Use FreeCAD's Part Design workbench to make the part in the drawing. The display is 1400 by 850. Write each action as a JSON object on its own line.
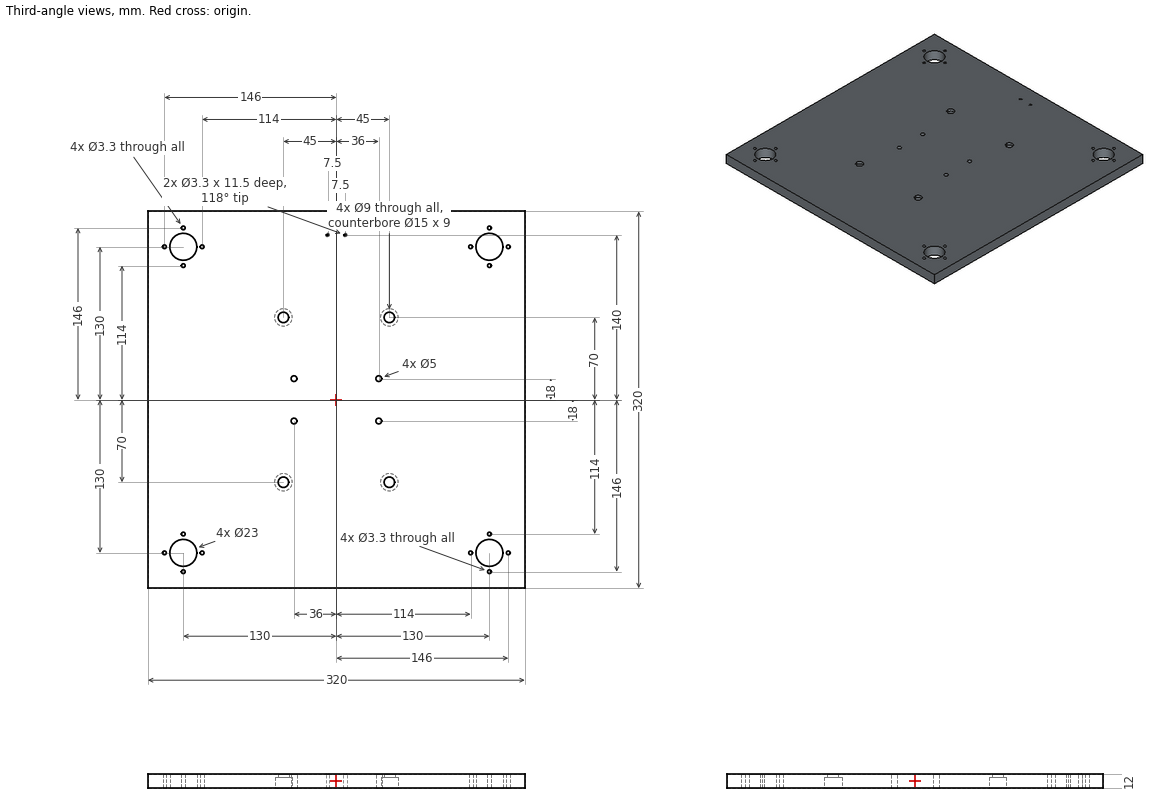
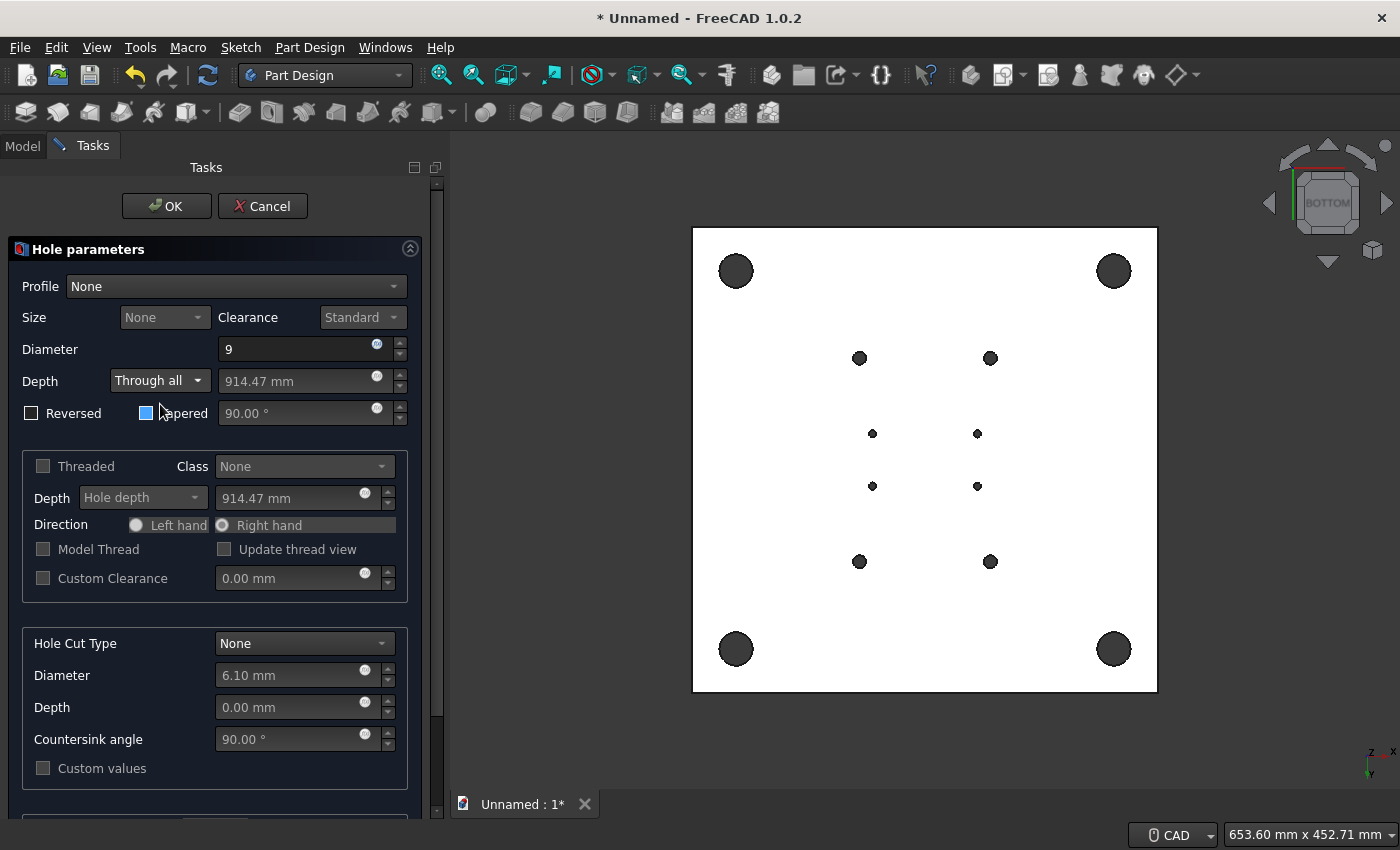
{"action": "left_click", "coordinate": [306, 644]}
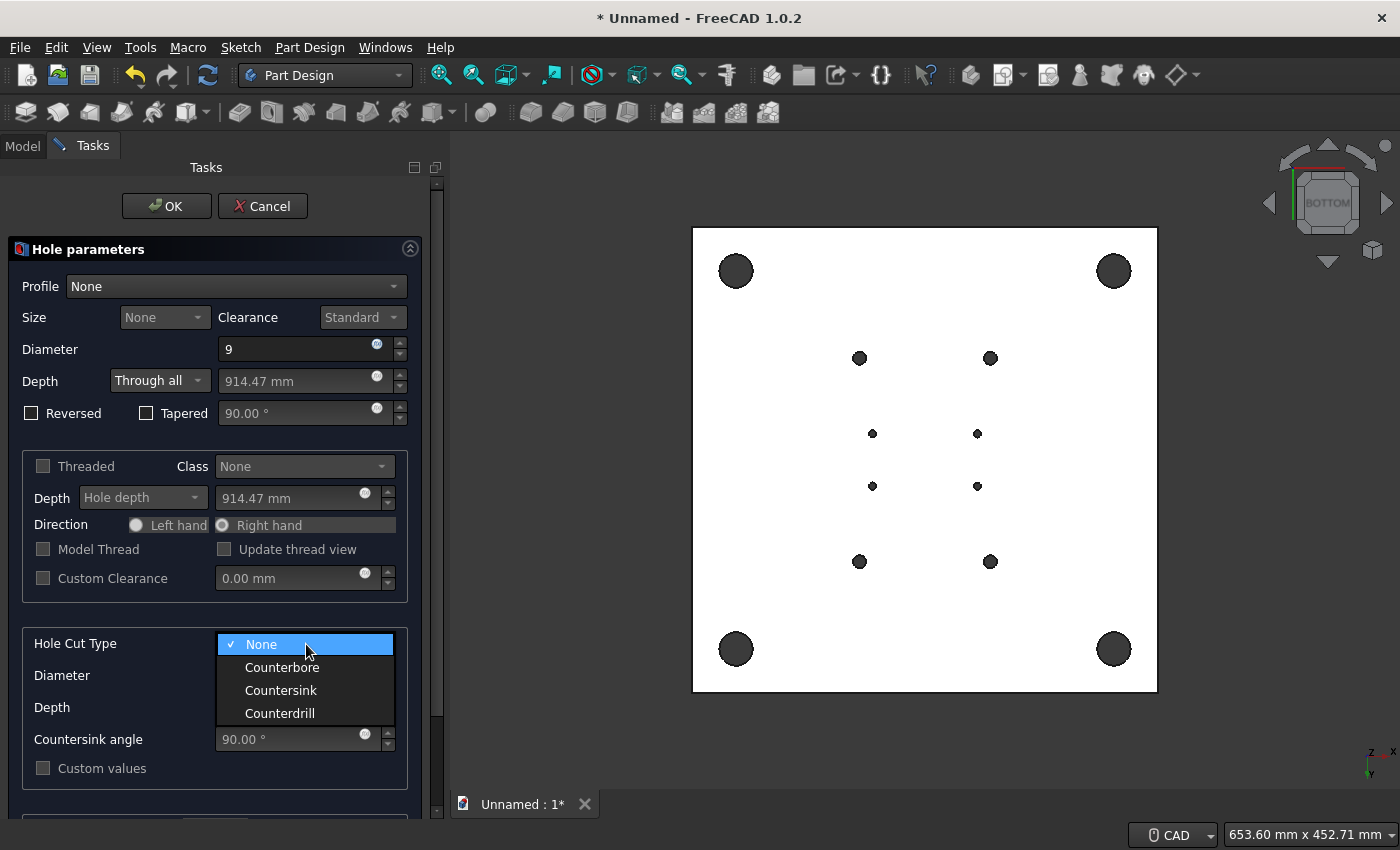
{"action": "left_click", "coordinate": [304, 668]}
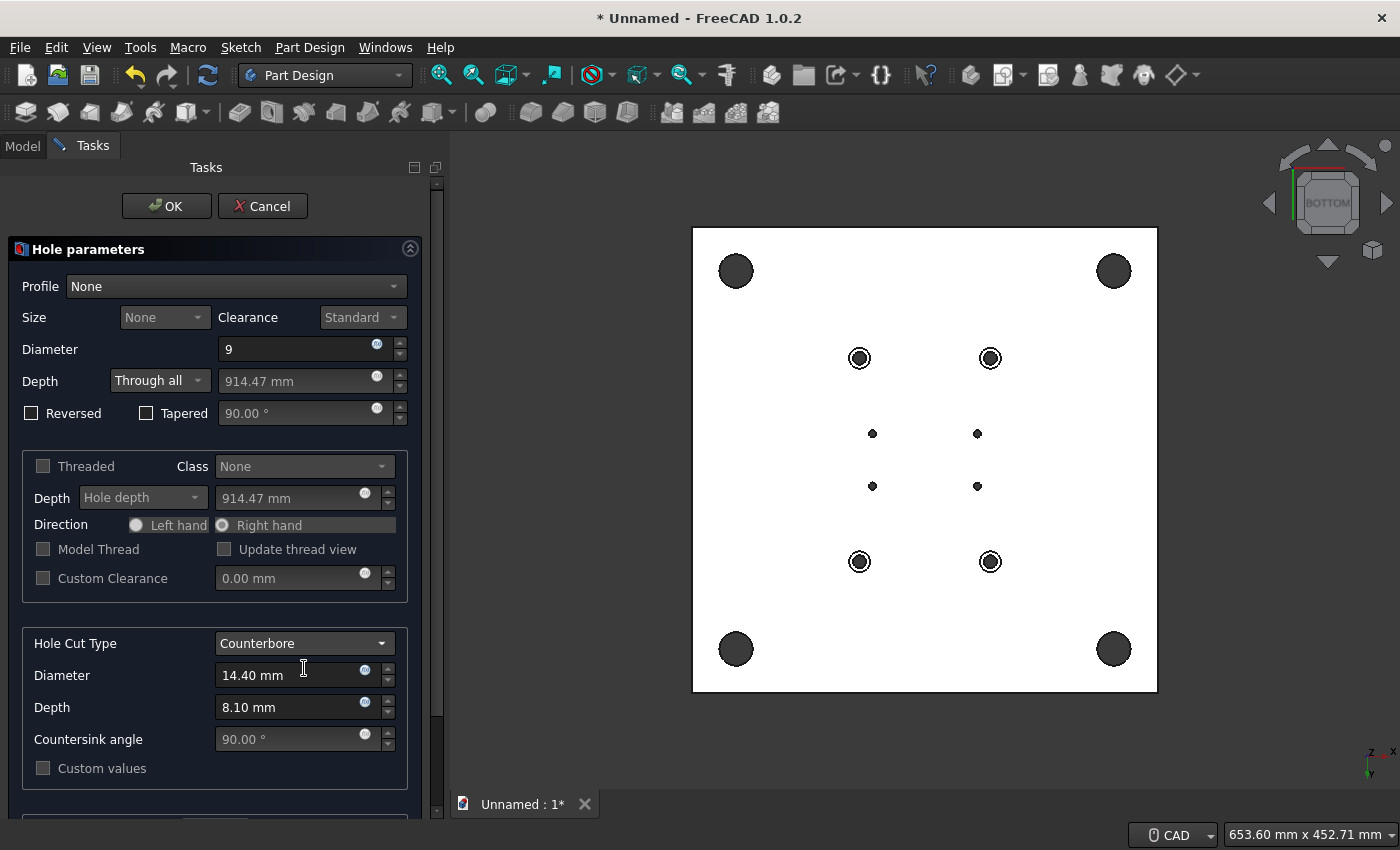
{"action": "triple_click", "coordinate": [298, 675]}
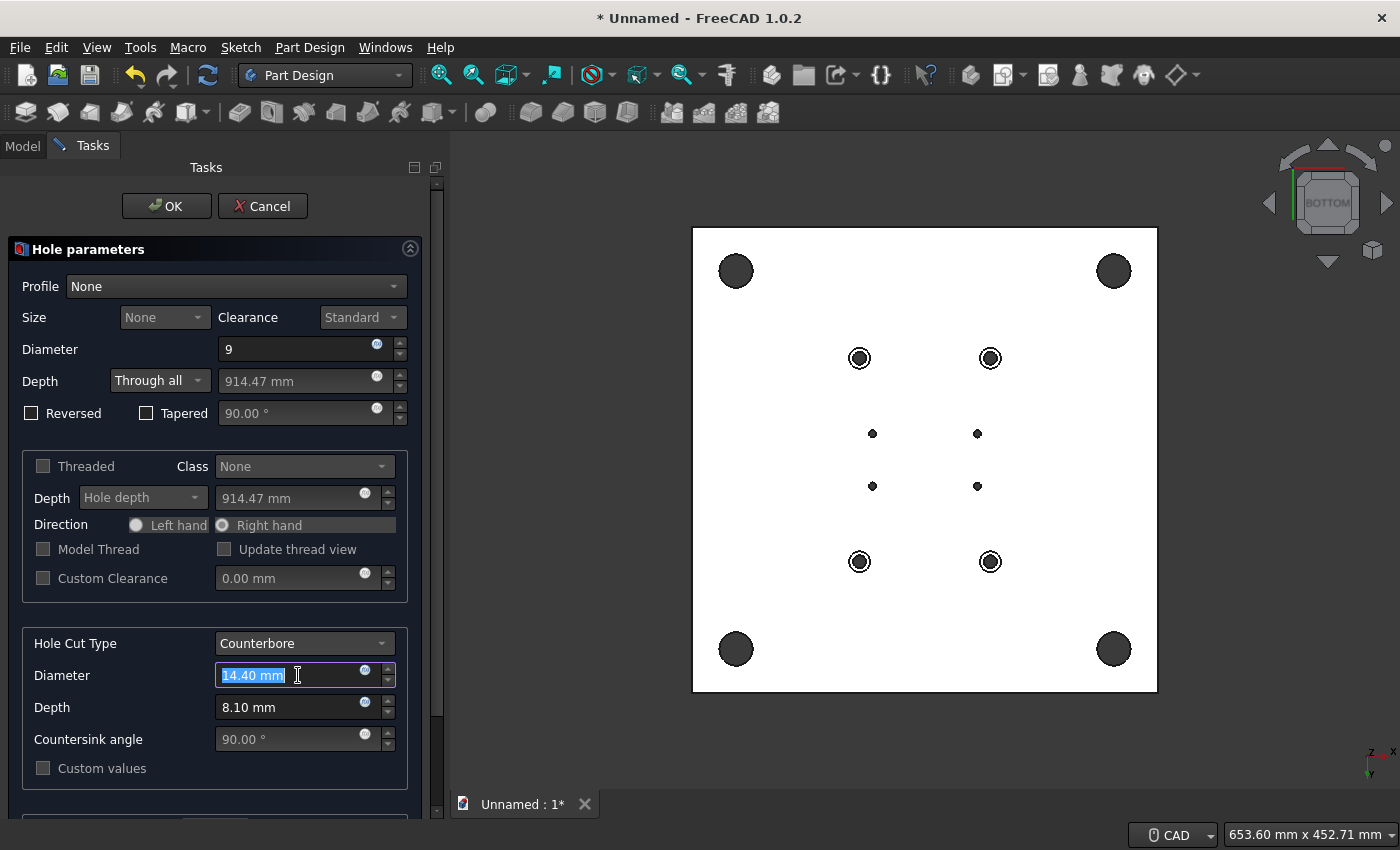
{"action": "type", "text": "15"}
{"action": "key", "text": "Tab"}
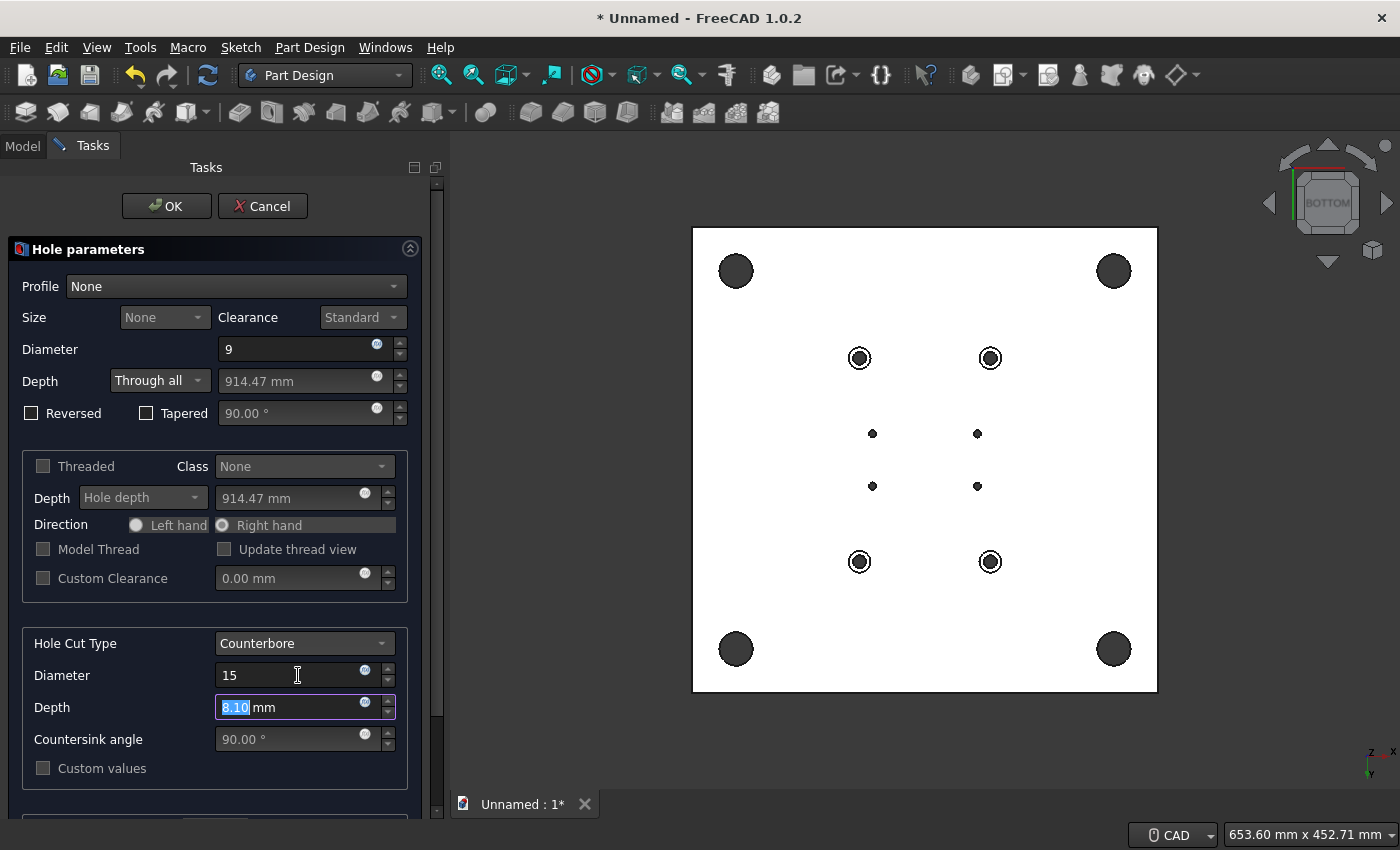
{"action": "type", "text": "9"}
{"action": "key", "text": "Tab"}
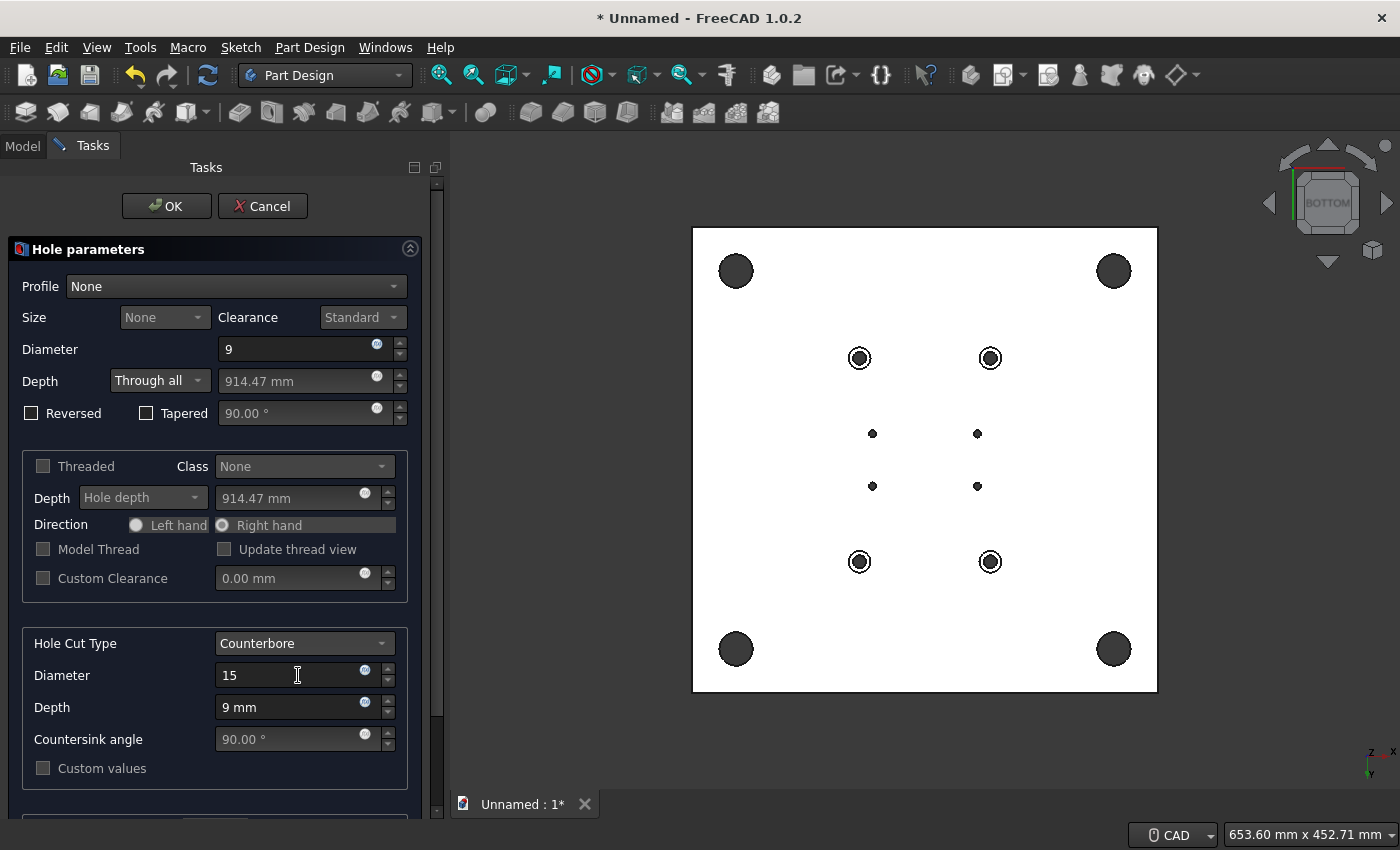
{"action": "left_click", "coordinate": [167, 206]}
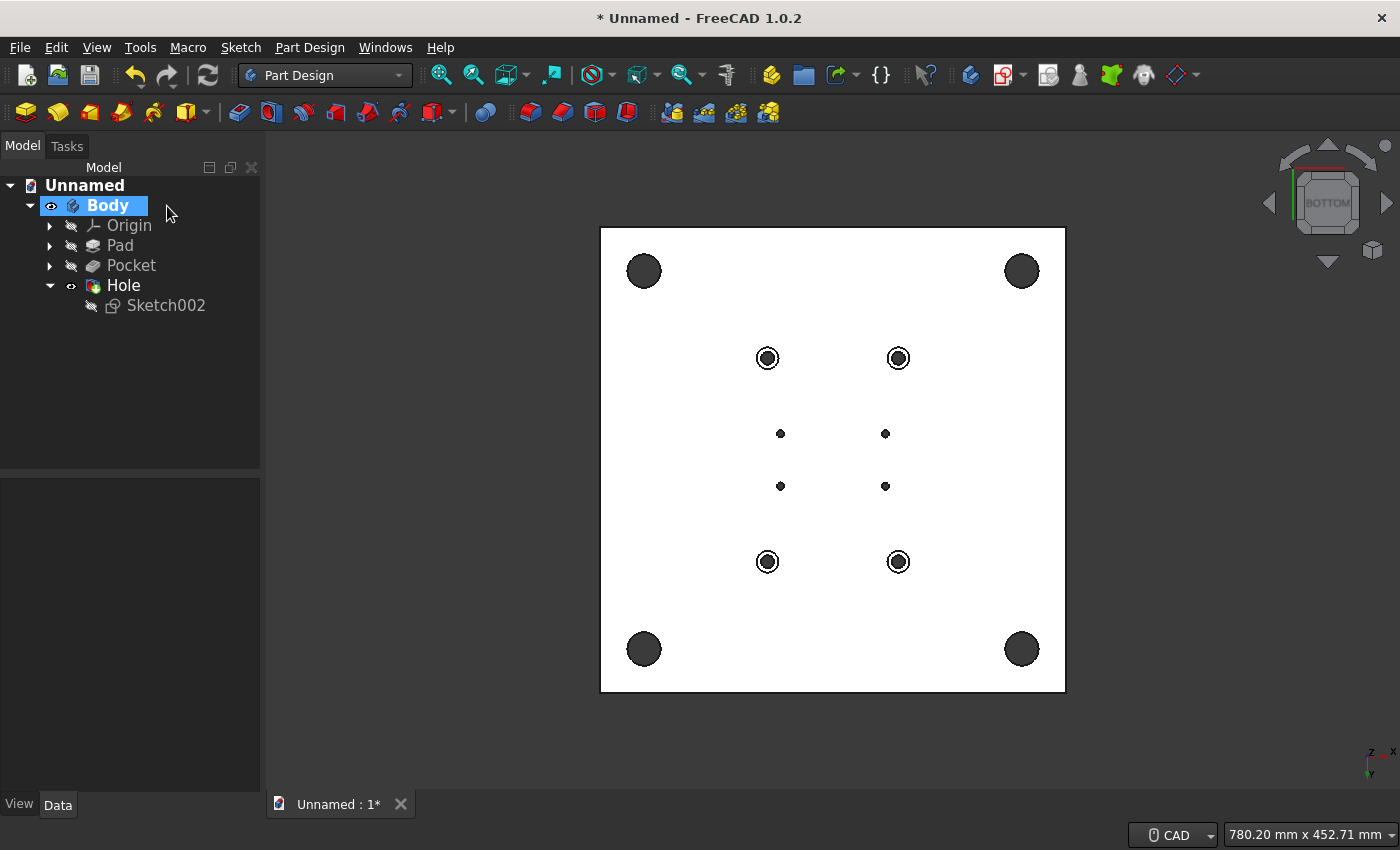
{"action": "key", "text": "0"}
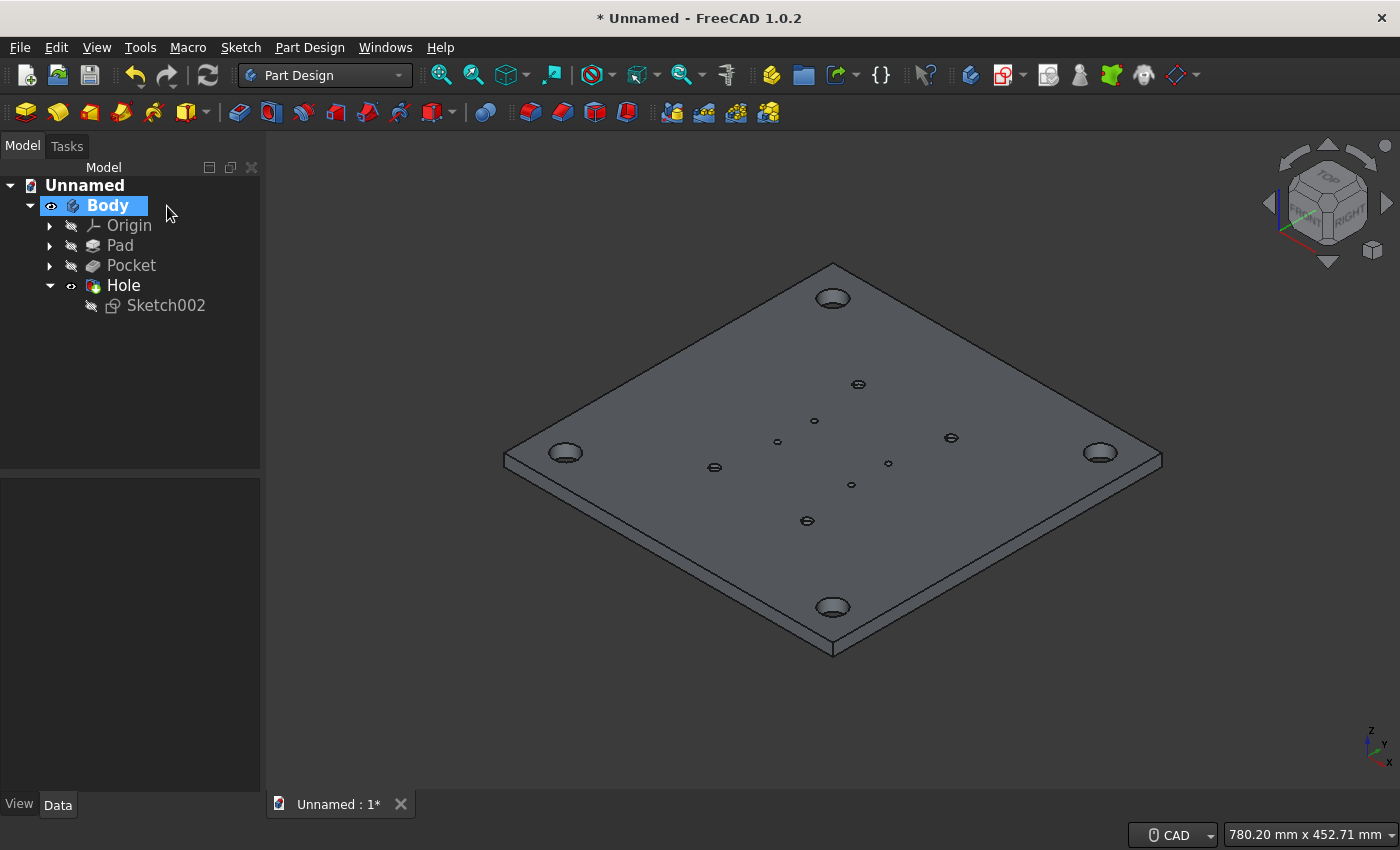
{"action": "left_click", "coordinate": [739, 398]}